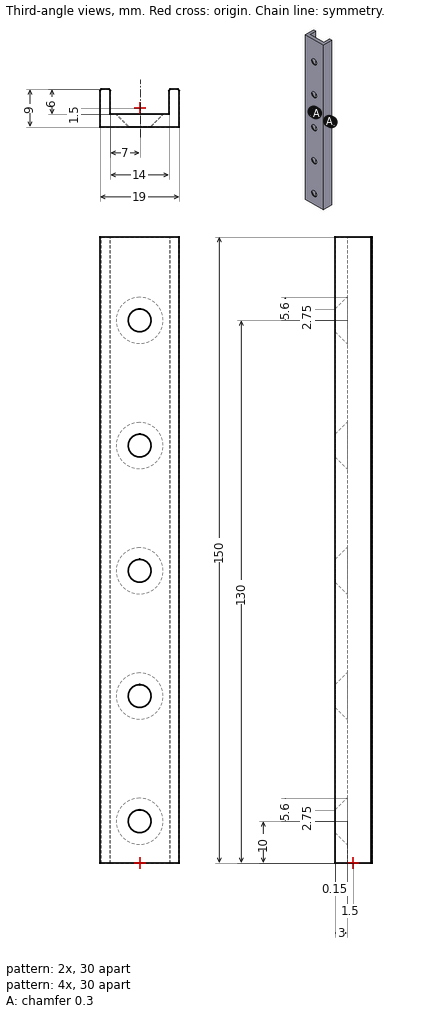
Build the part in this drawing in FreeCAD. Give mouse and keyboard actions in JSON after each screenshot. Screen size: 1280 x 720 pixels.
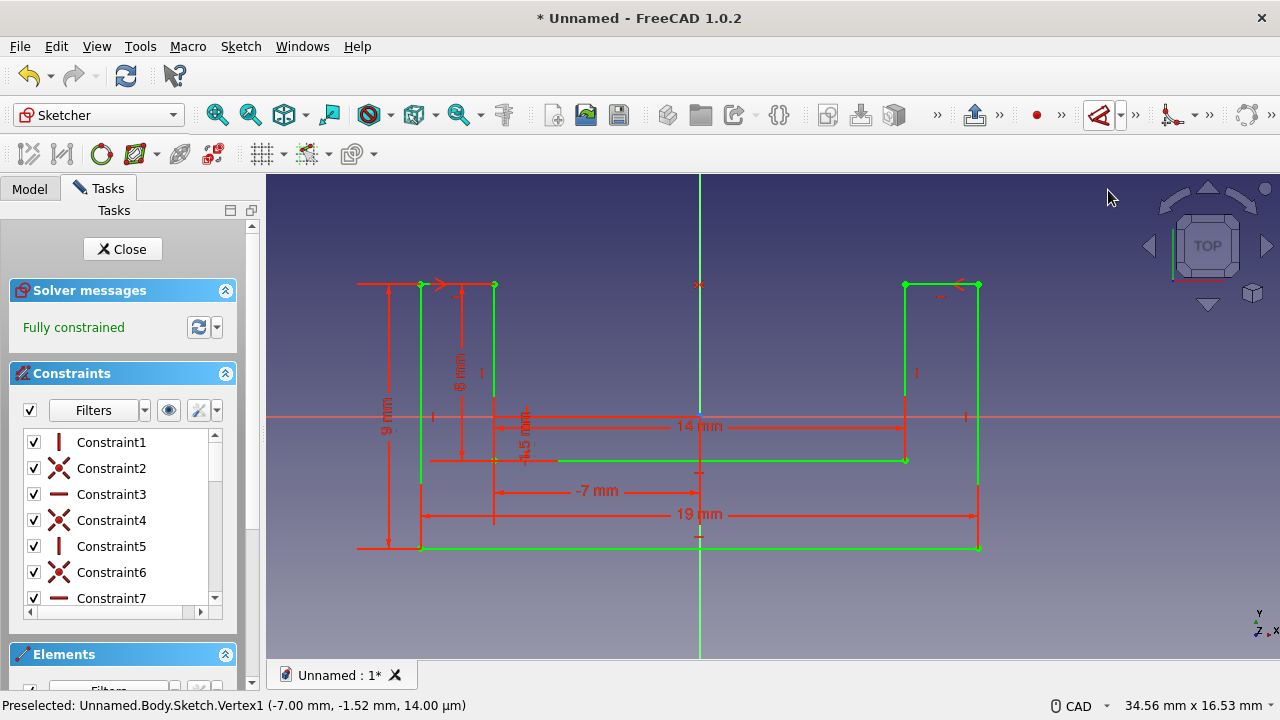
{"action": "left_click", "coordinate": [123, 249]}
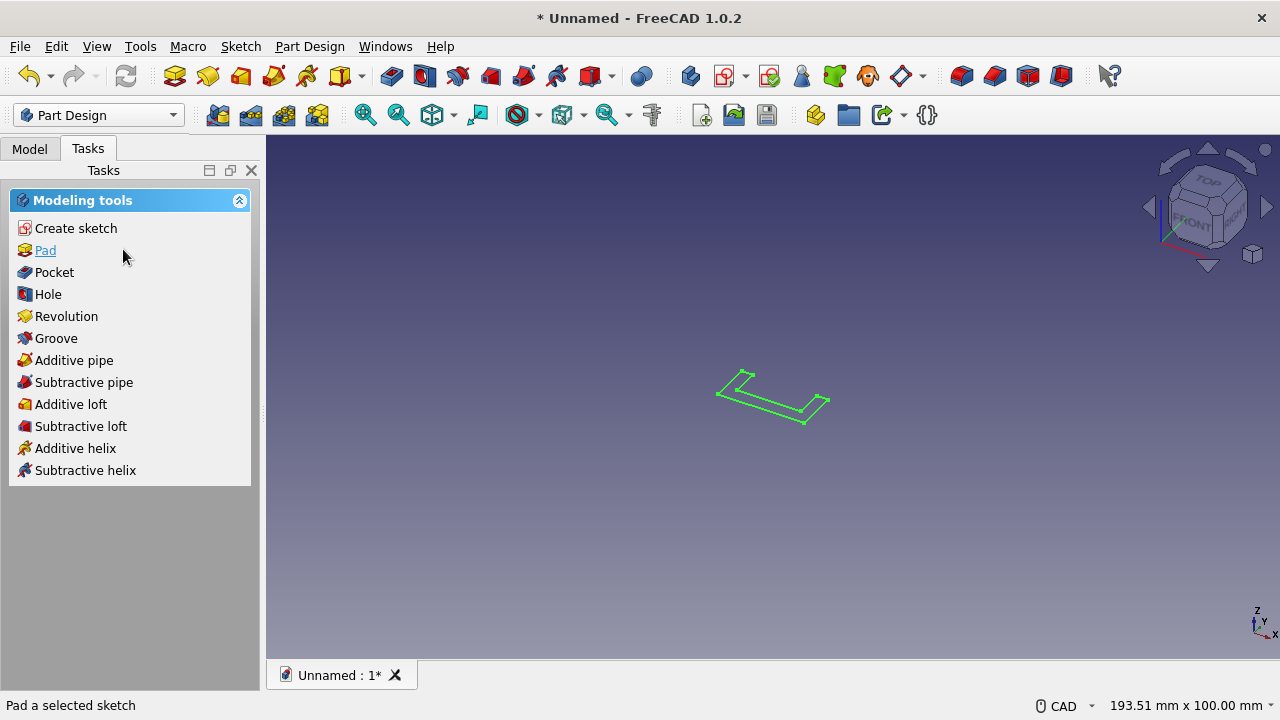
{"action": "left_click", "coordinate": [175, 76]}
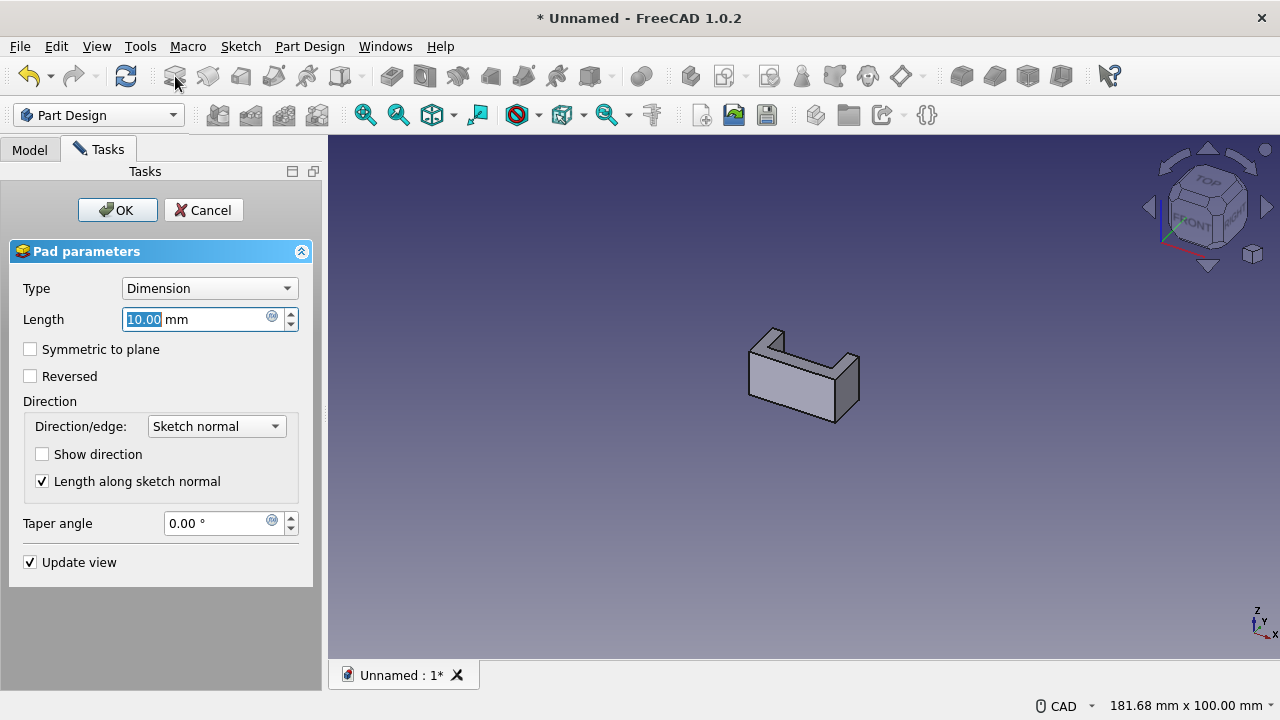
{"action": "type", "text": "150"}
{"action": "key", "text": "Tab"}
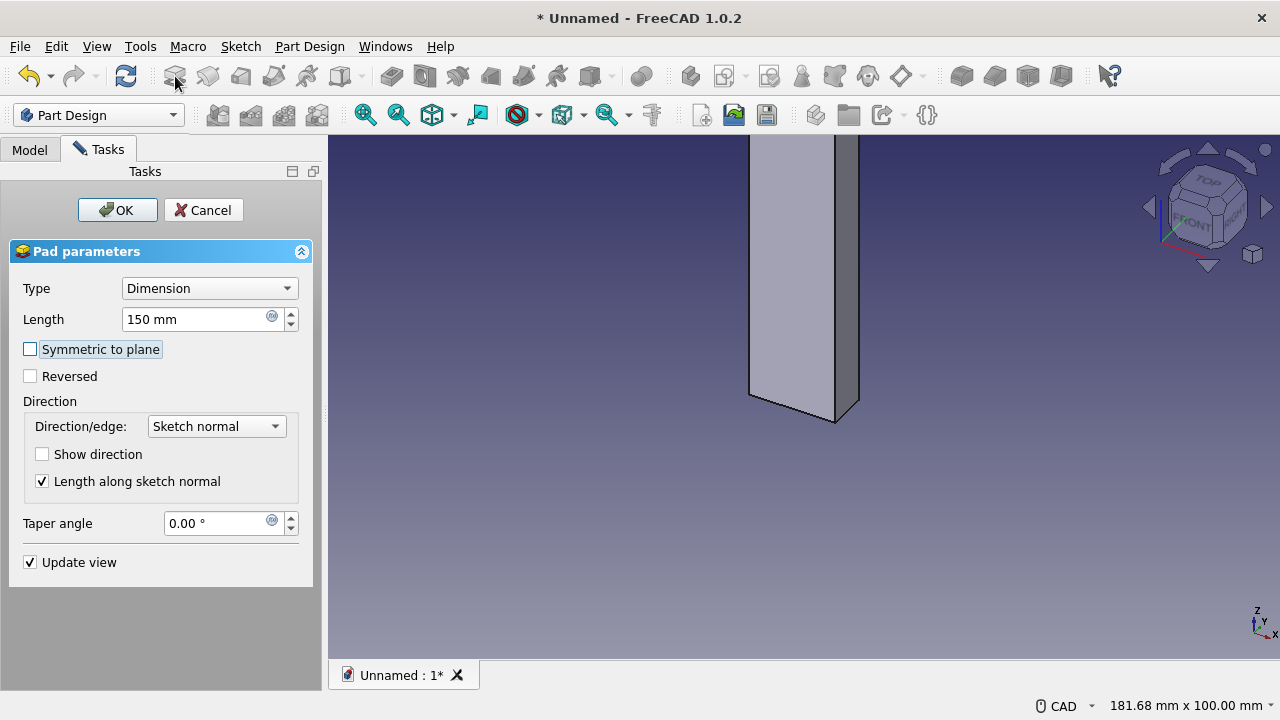
{"action": "left_click", "coordinate": [118, 210]}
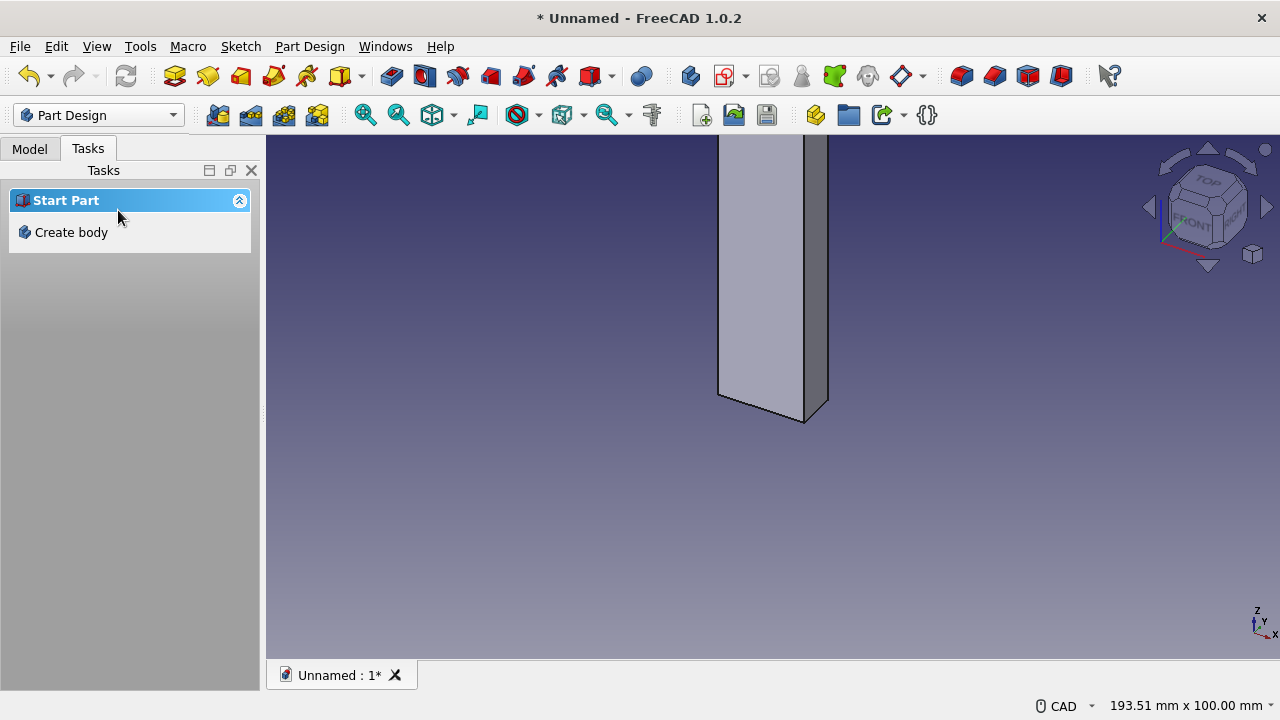
{"action": "left_click", "coordinate": [366, 116]}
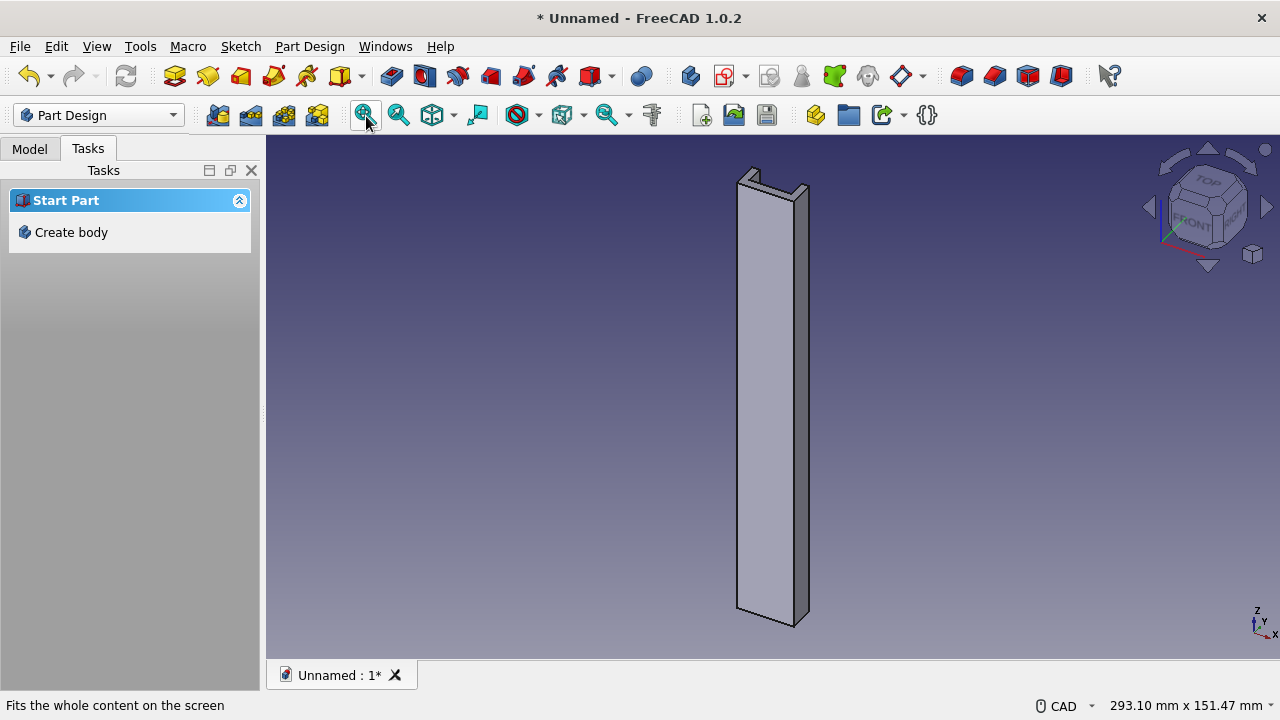
{"action": "left_click", "coordinate": [724, 76]}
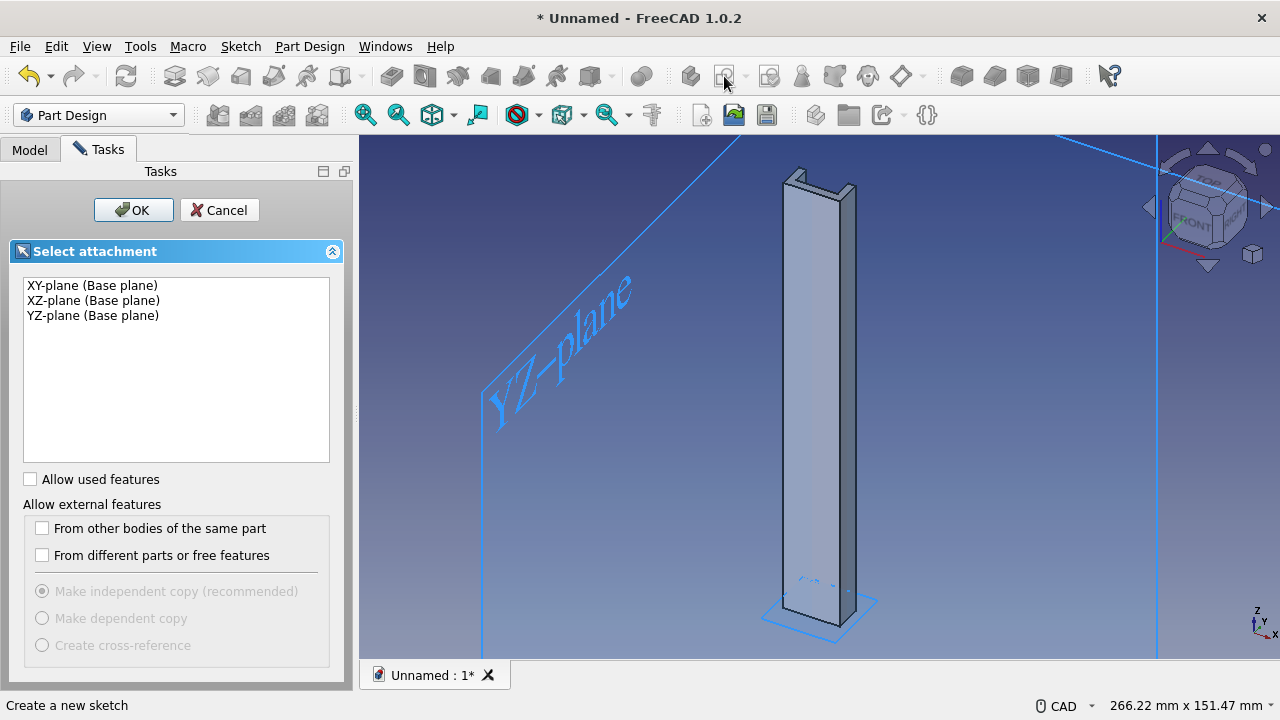
{"action": "left_click", "coordinate": [84, 316]}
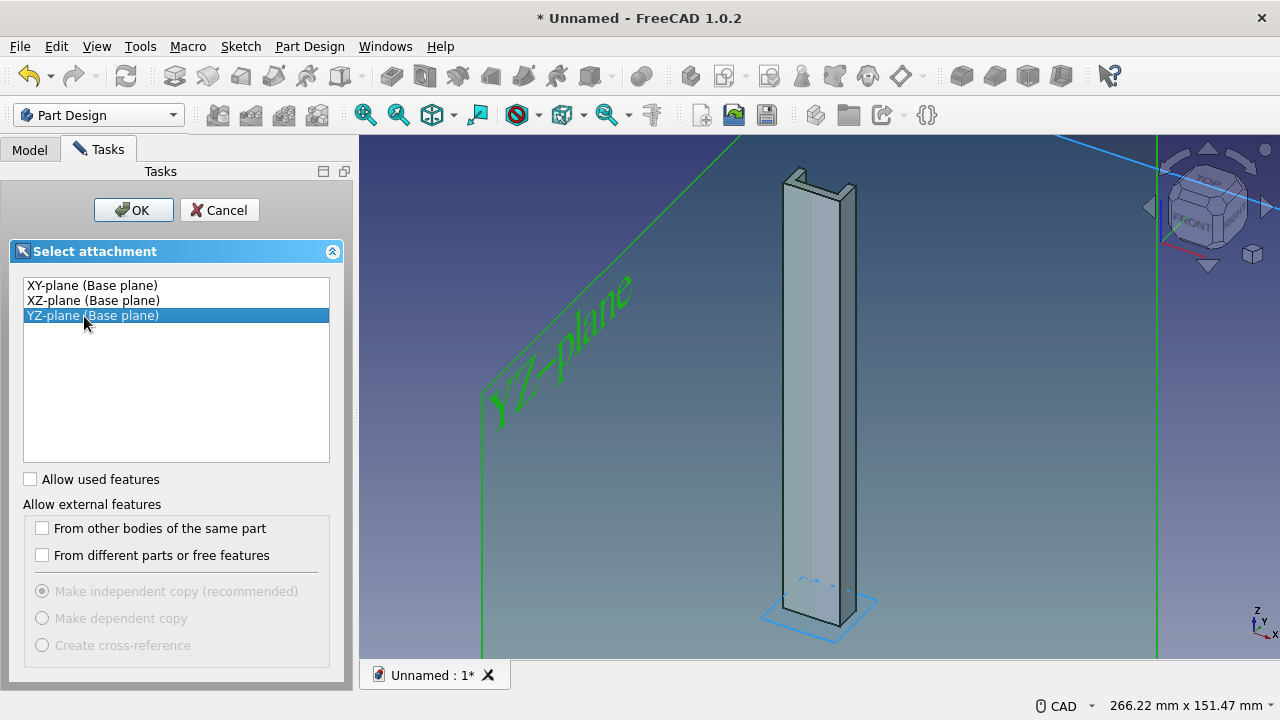
{"action": "left_click", "coordinate": [134, 210]}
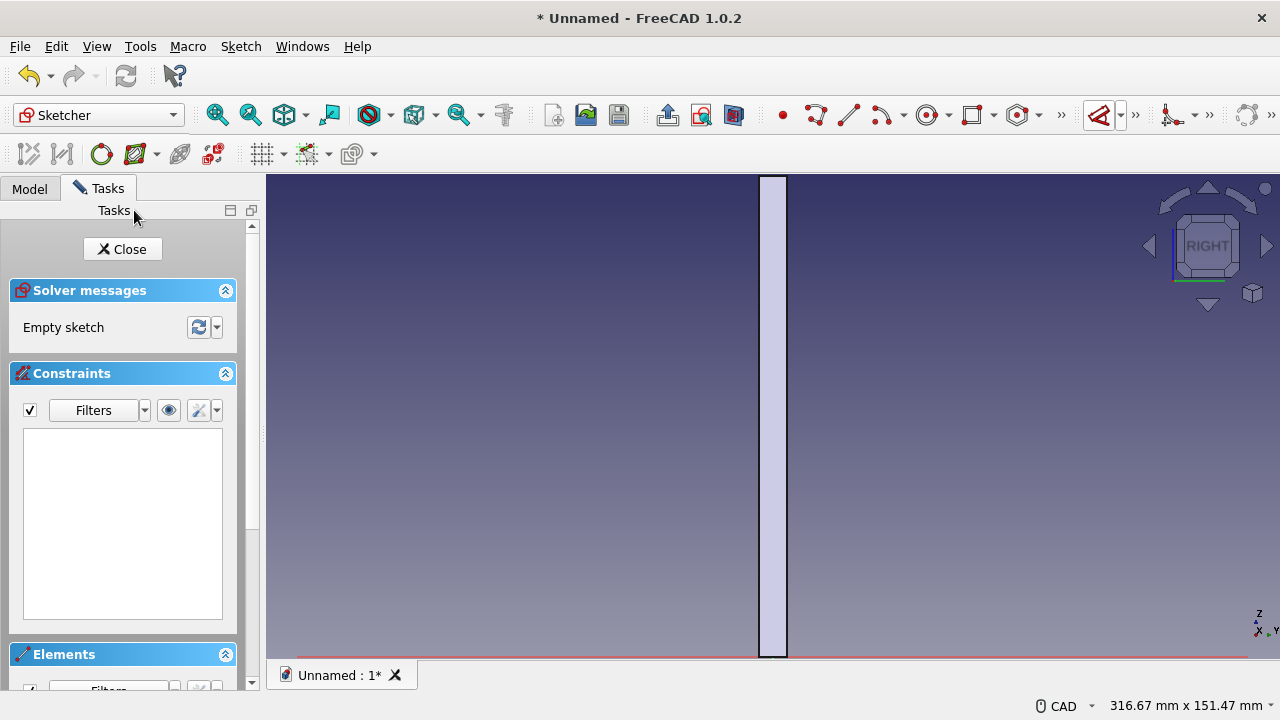
{"action": "left_click", "coordinate": [734, 116]}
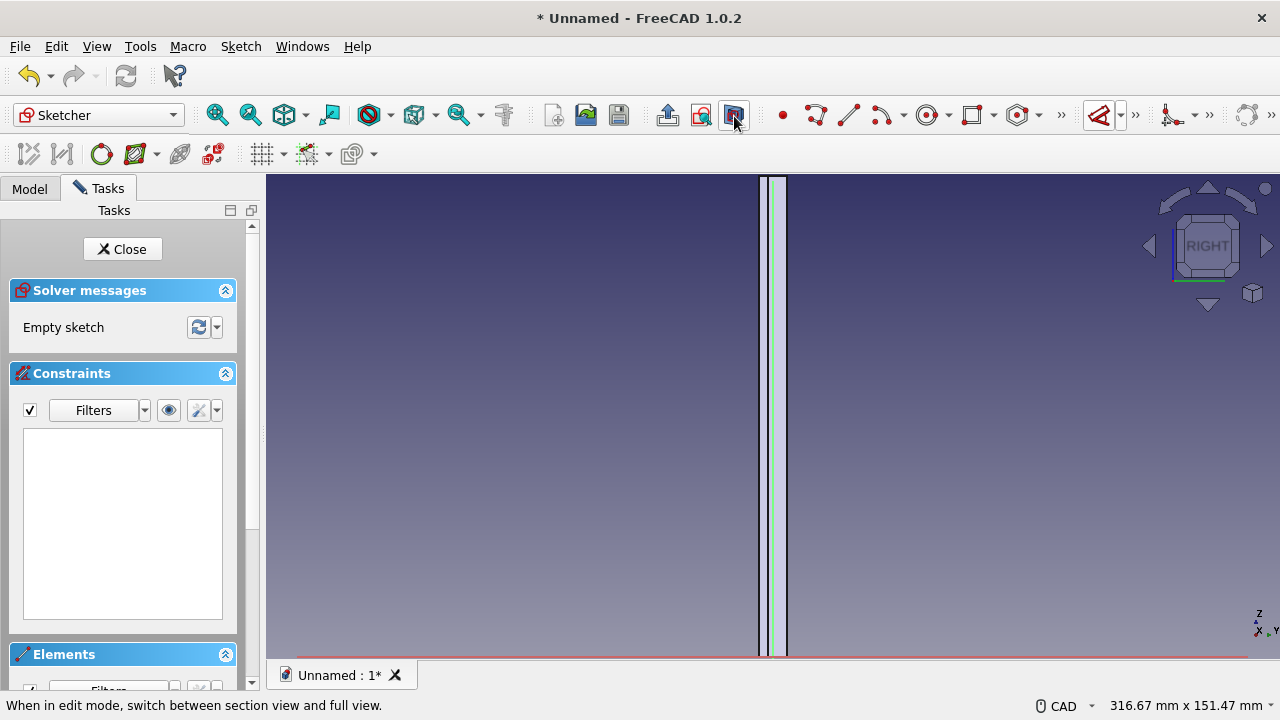
{"action": "scroll", "coordinate": [765, 629], "scroll_direction": "up", "scroll_amount": 14}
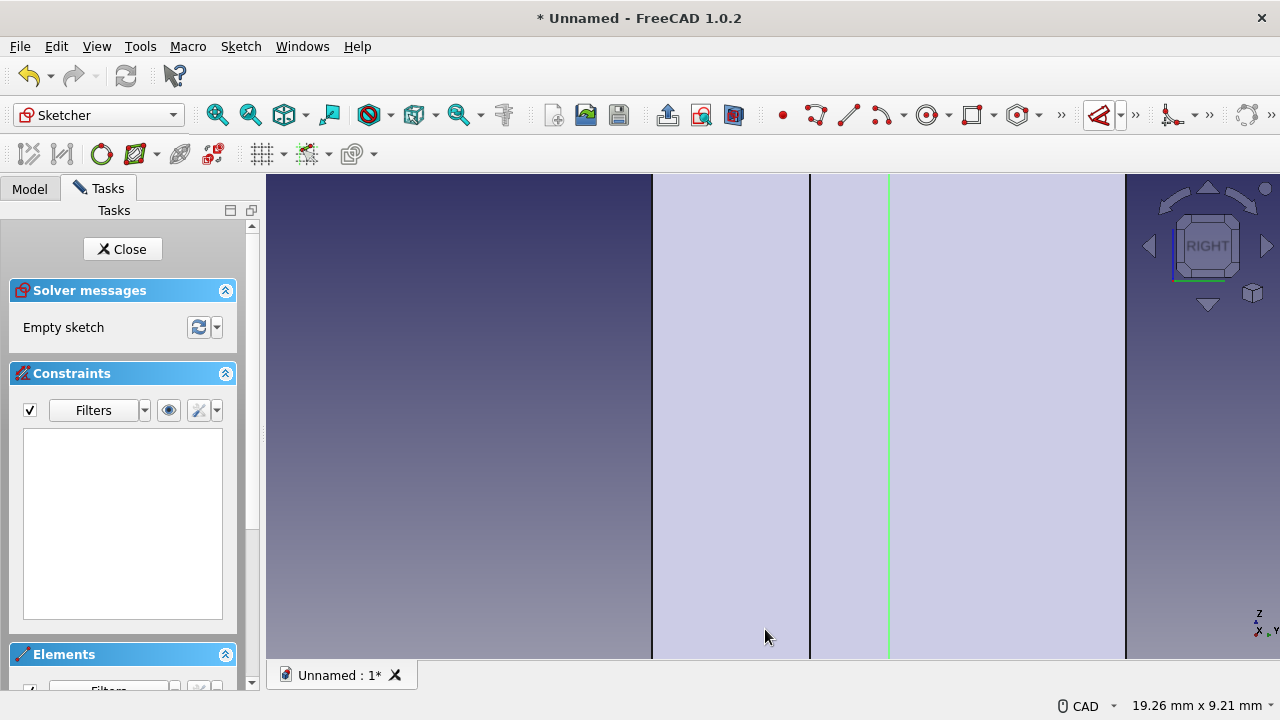
{"action": "left_click", "coordinate": [816, 116]}